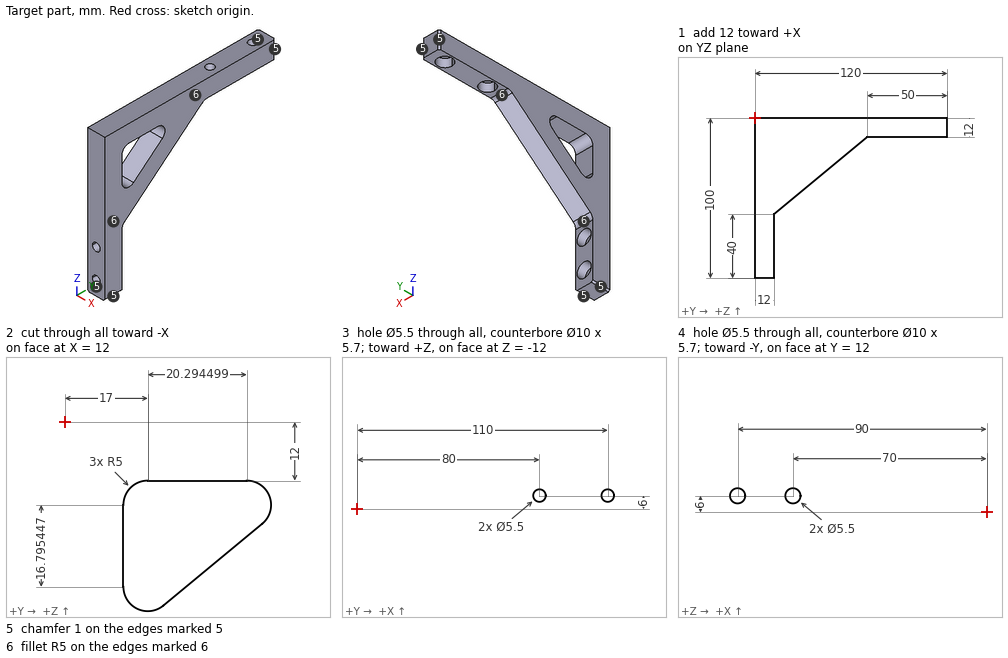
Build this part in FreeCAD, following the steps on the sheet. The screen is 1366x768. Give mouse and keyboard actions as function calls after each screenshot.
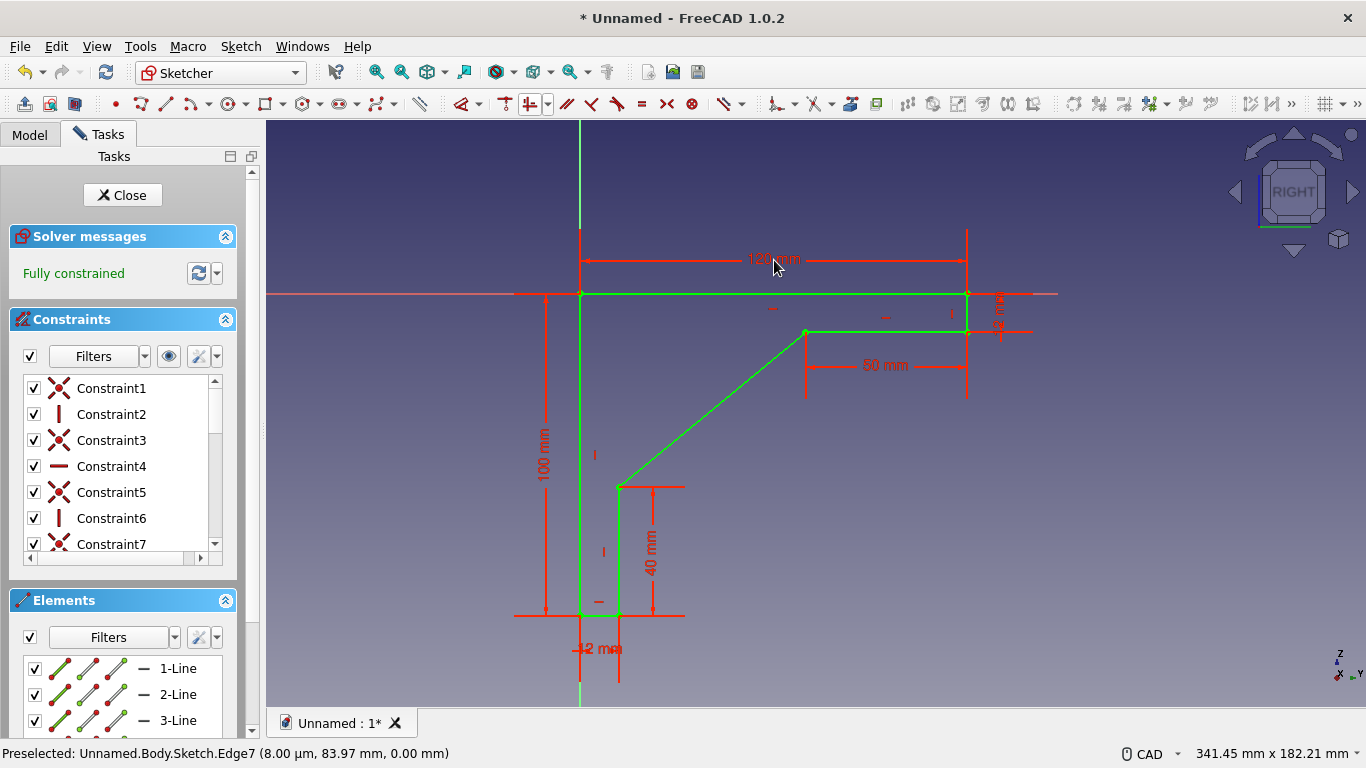
click(123, 195)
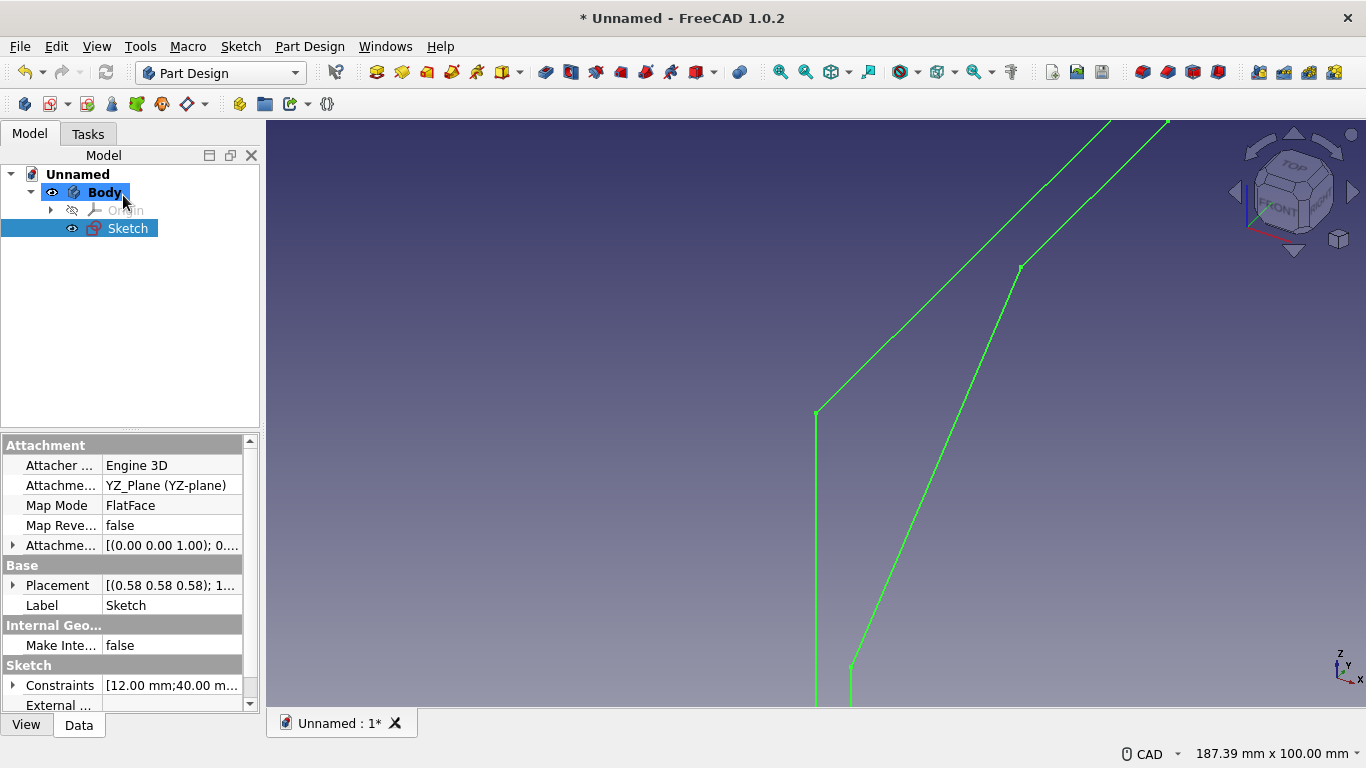
click(377, 72)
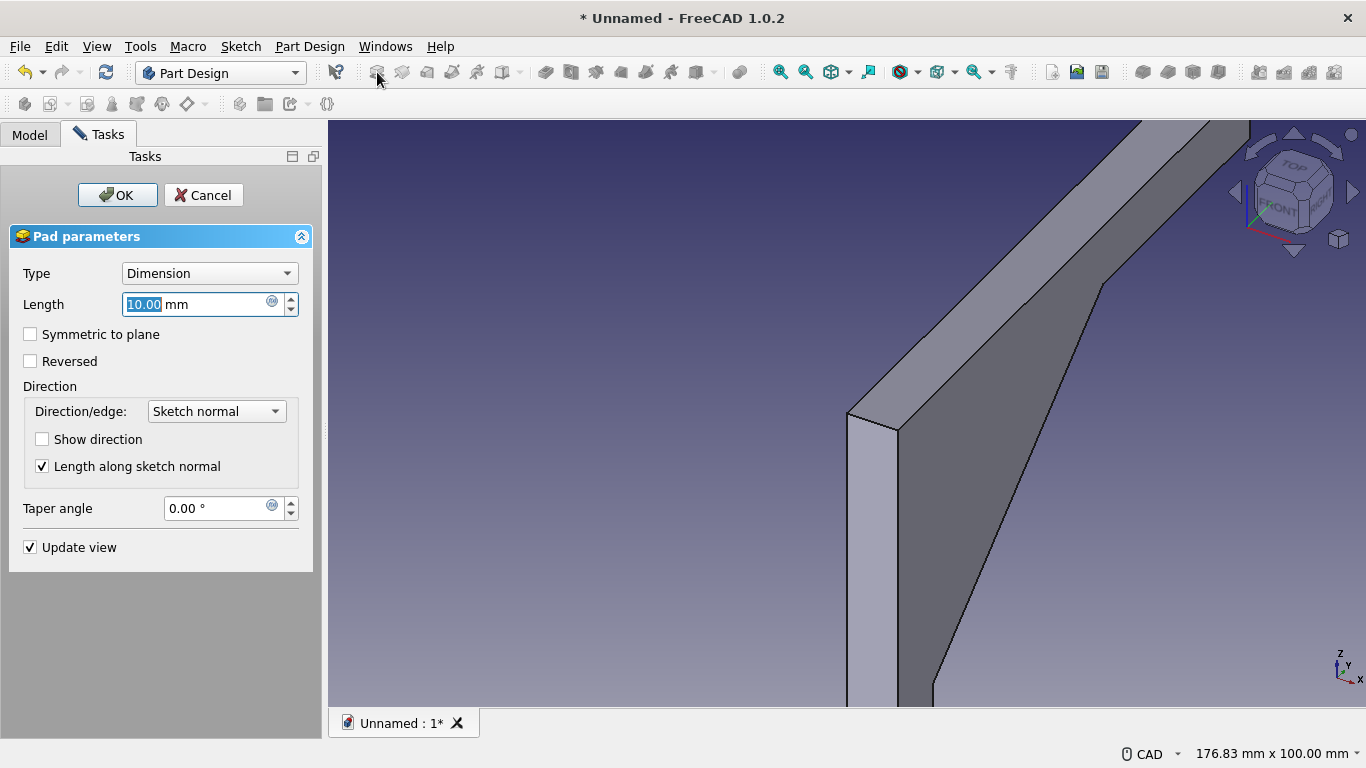
text(12)
key(Tab)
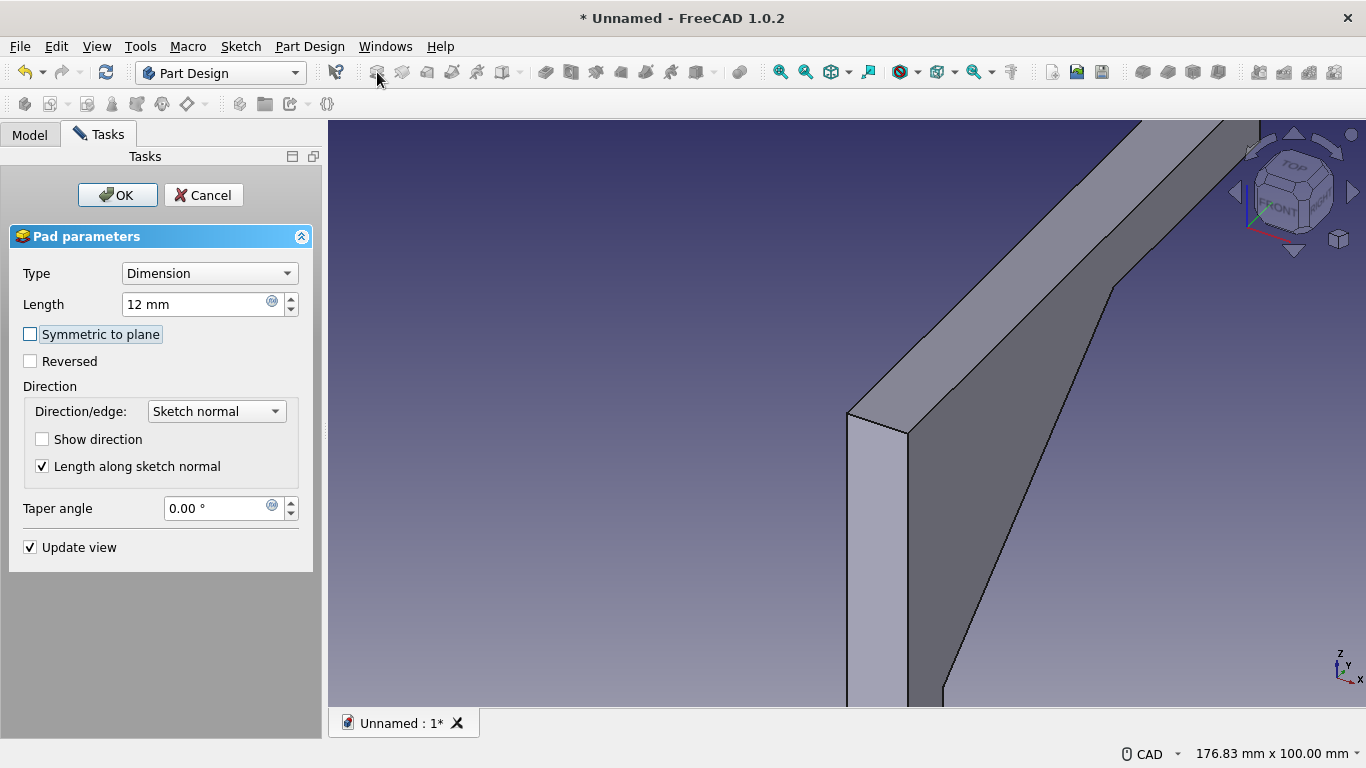
click(118, 195)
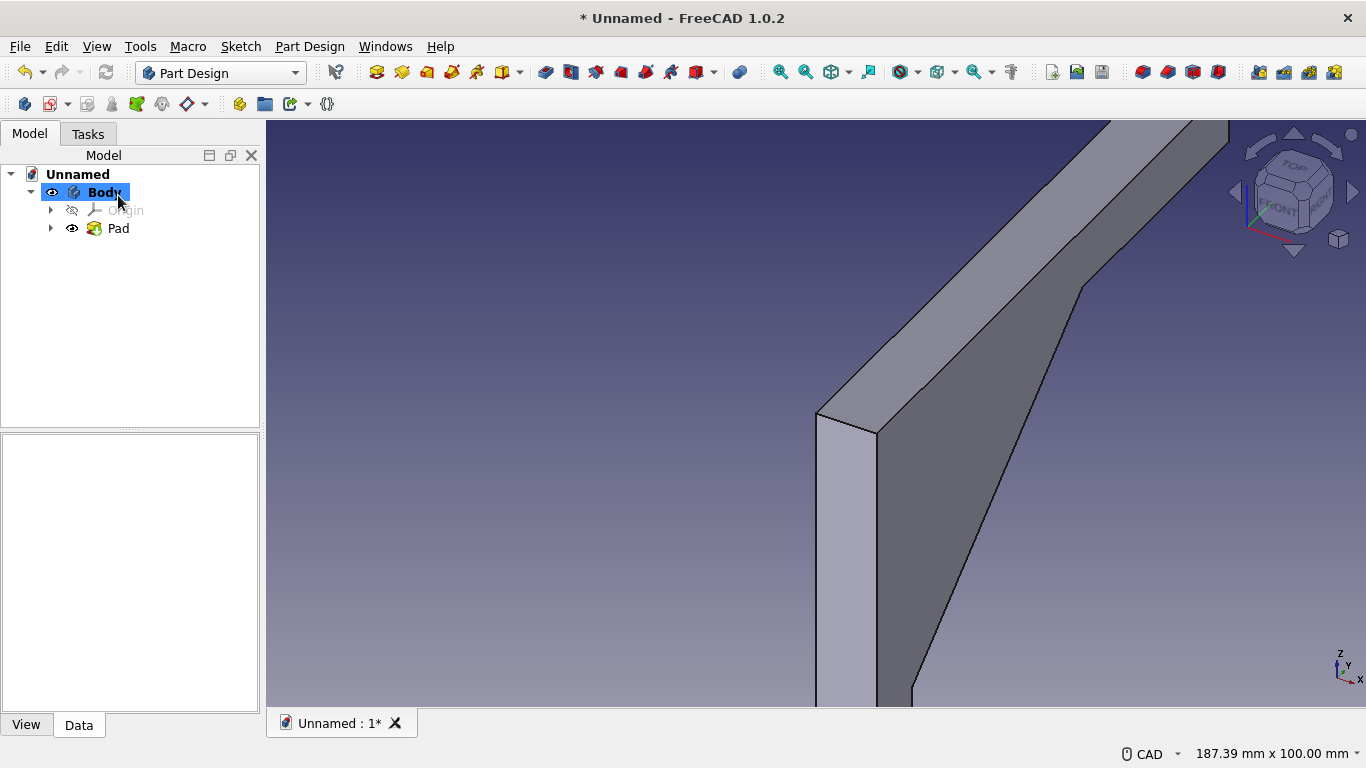
click(781, 72)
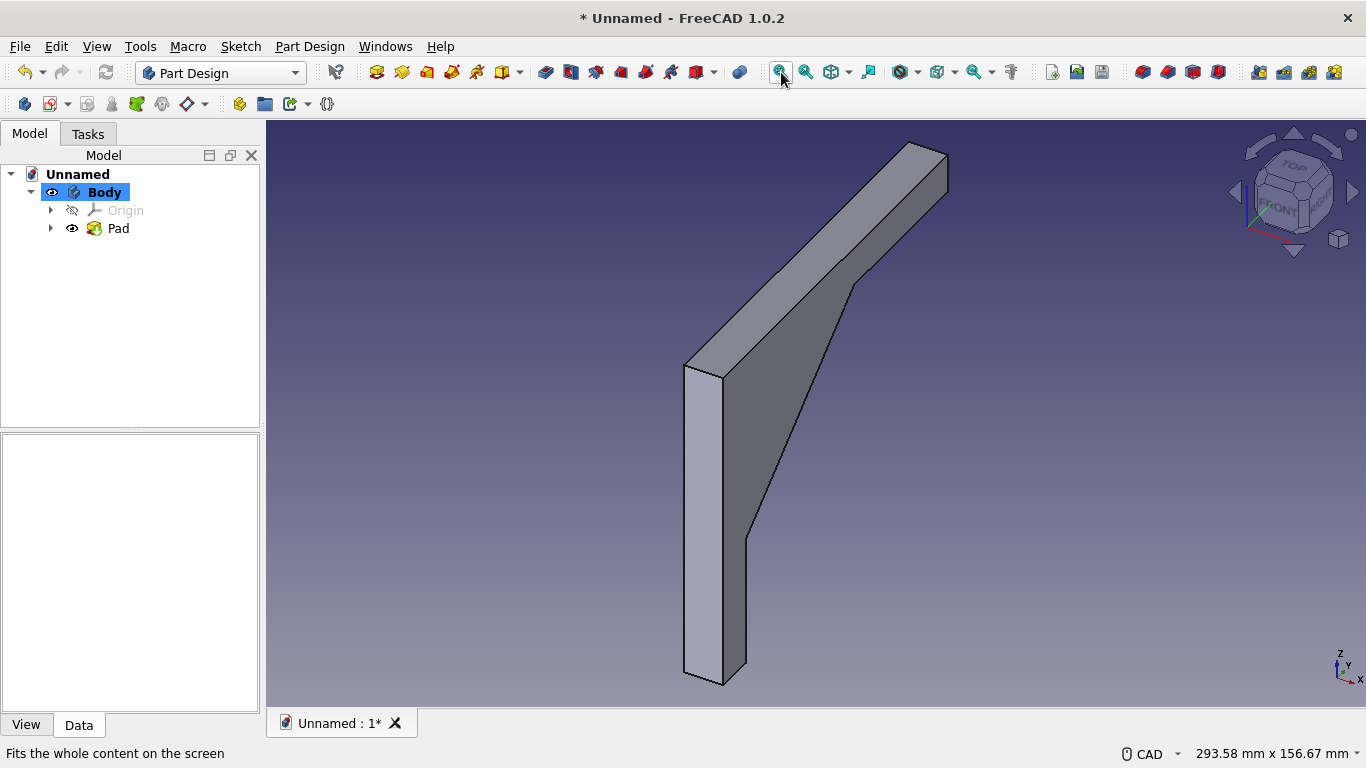
click(771, 395)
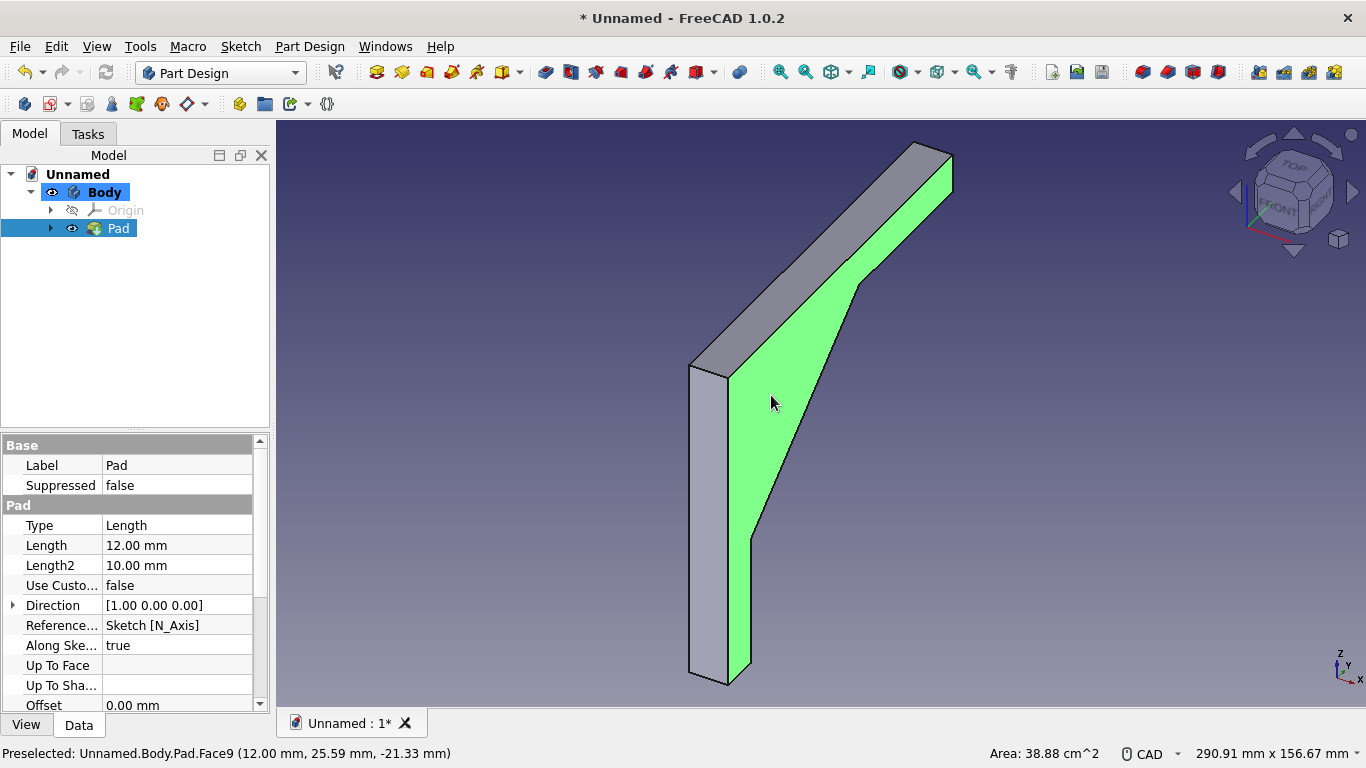
click(50, 104)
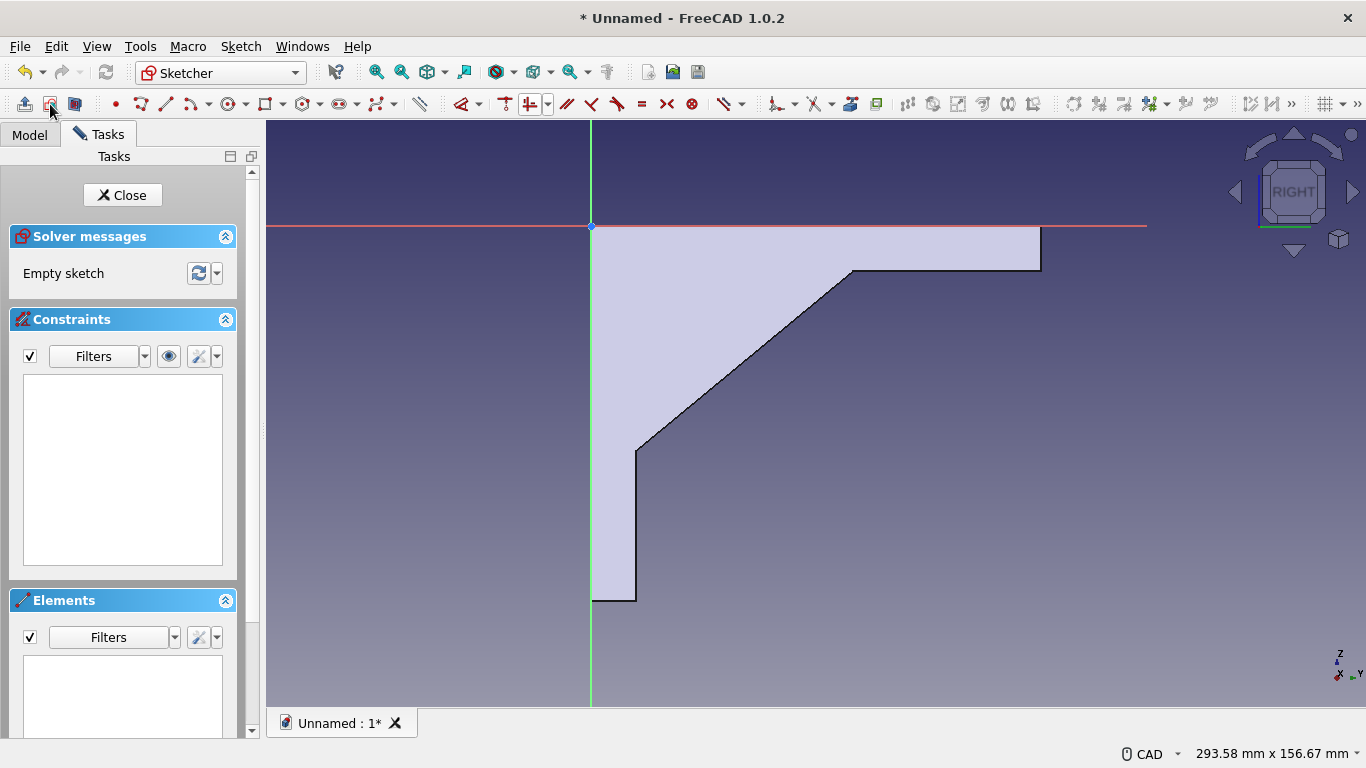
scroll(625, 231, up, 5)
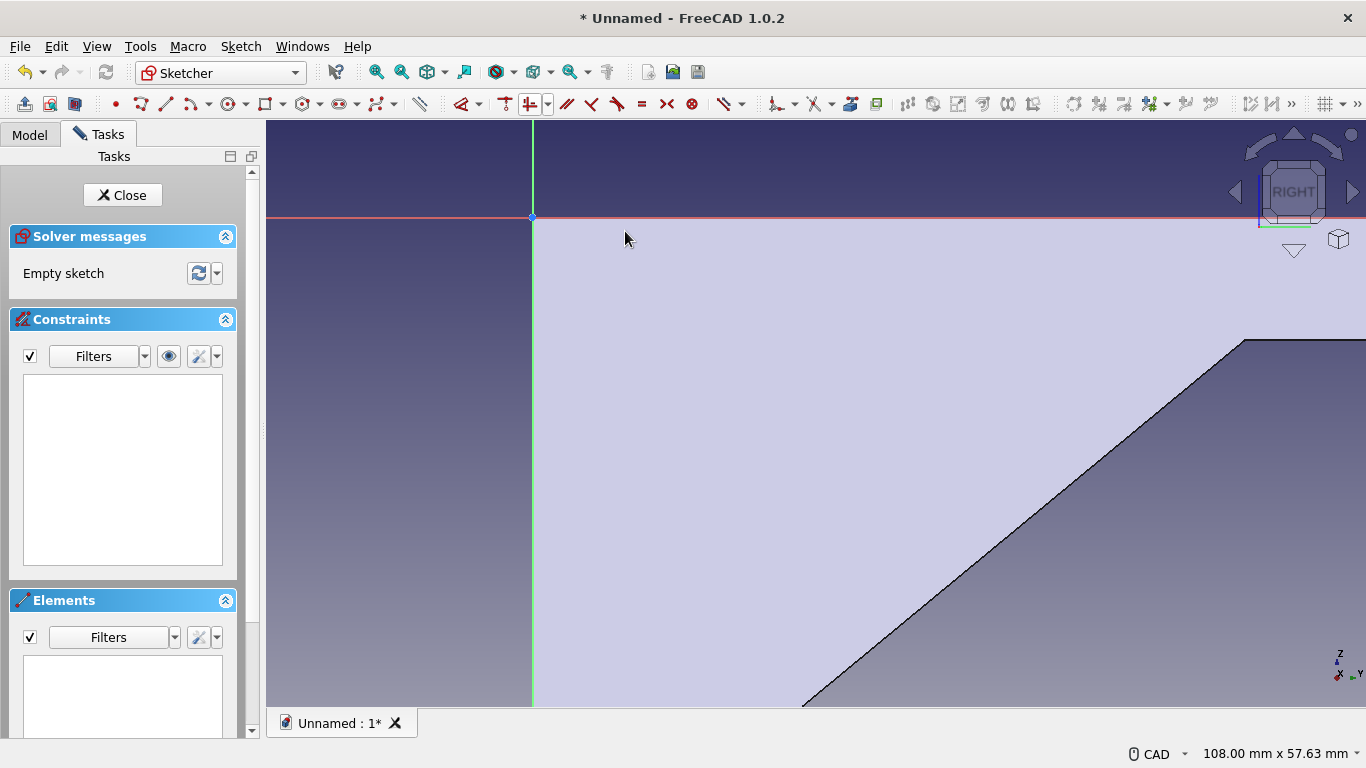
click(166, 104)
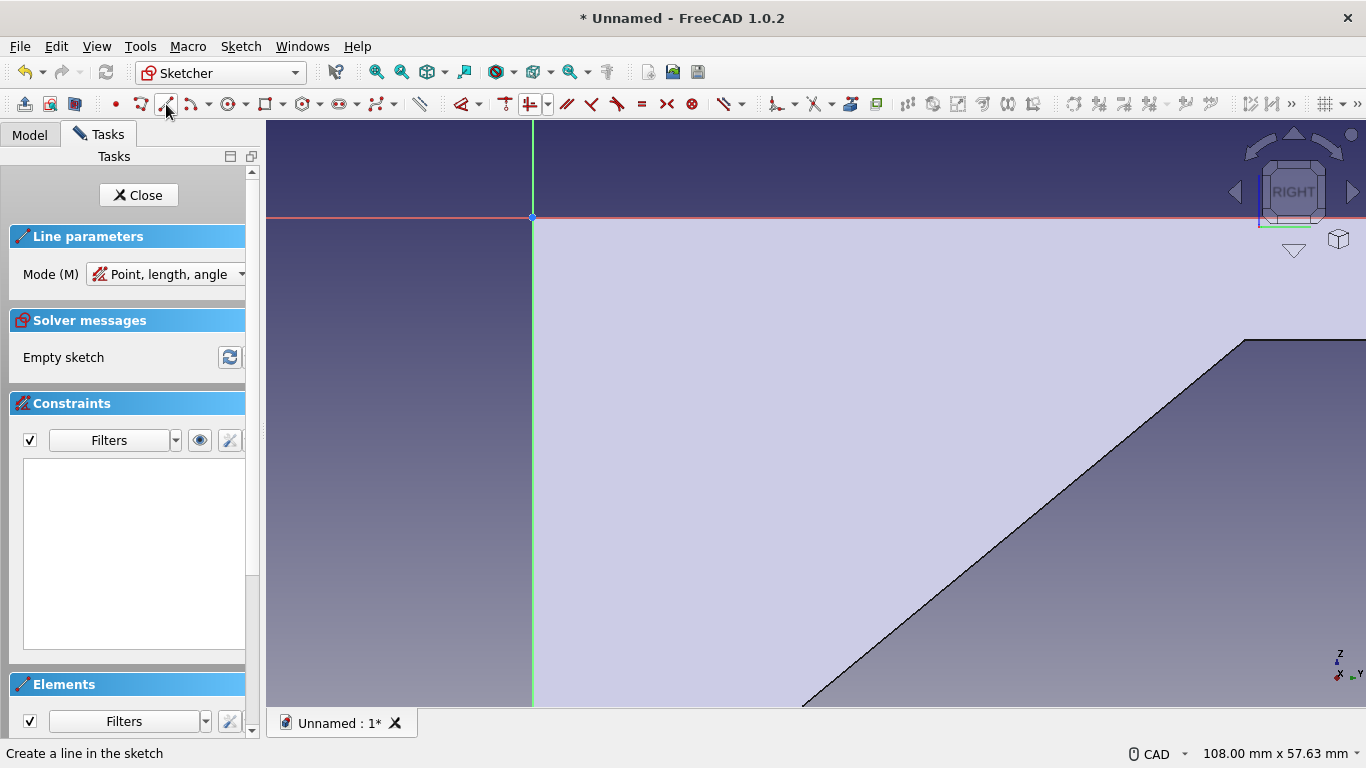
click(912, 340)
click(706, 340)